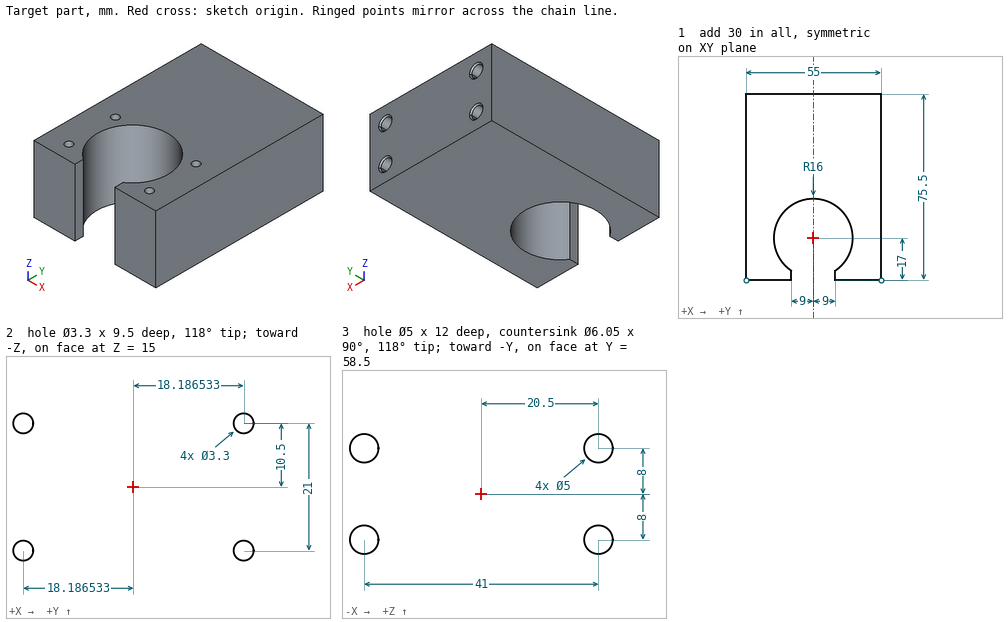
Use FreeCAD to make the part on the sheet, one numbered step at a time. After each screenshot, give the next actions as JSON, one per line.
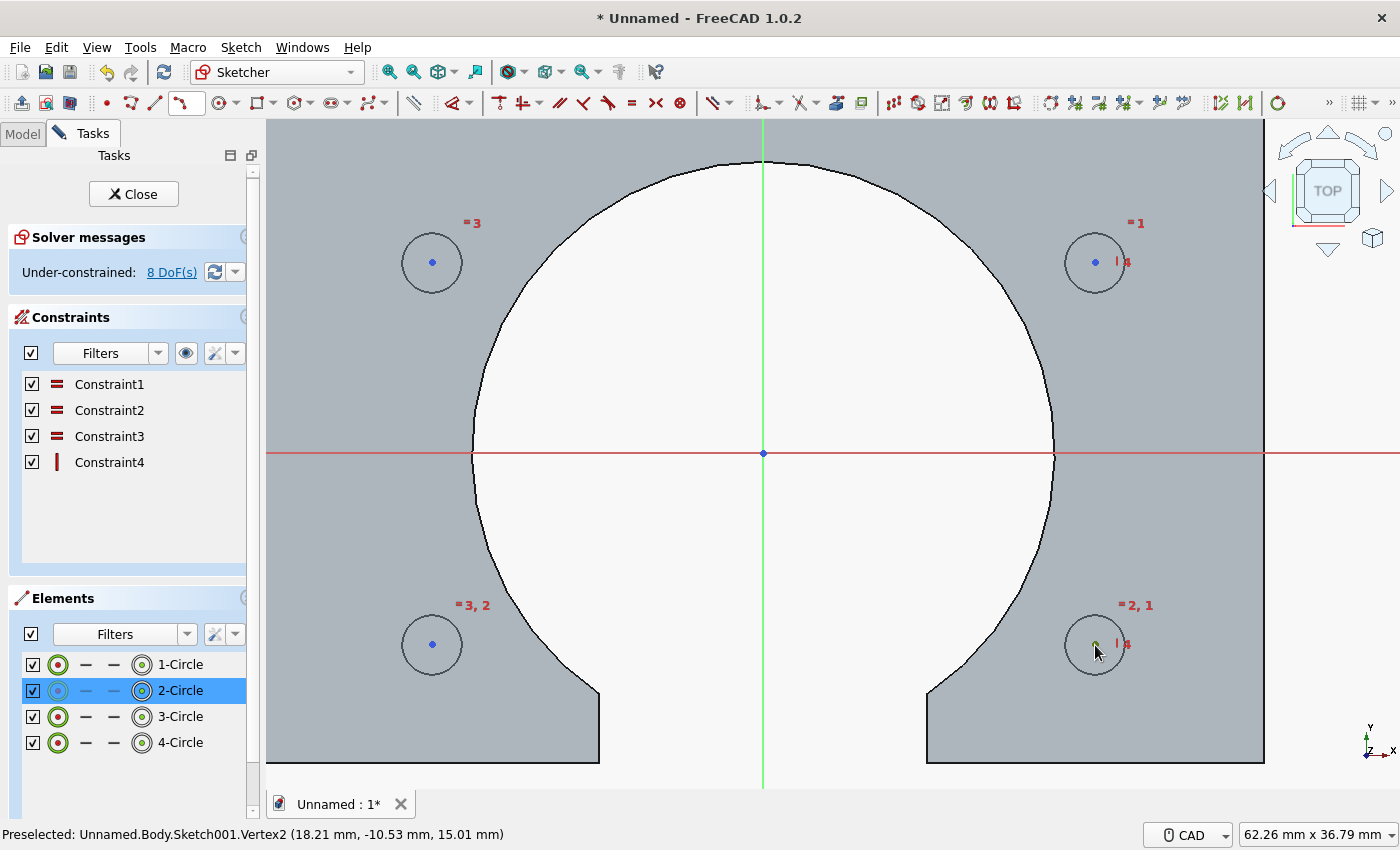
{"action": "left_click", "coordinate": [432, 645]}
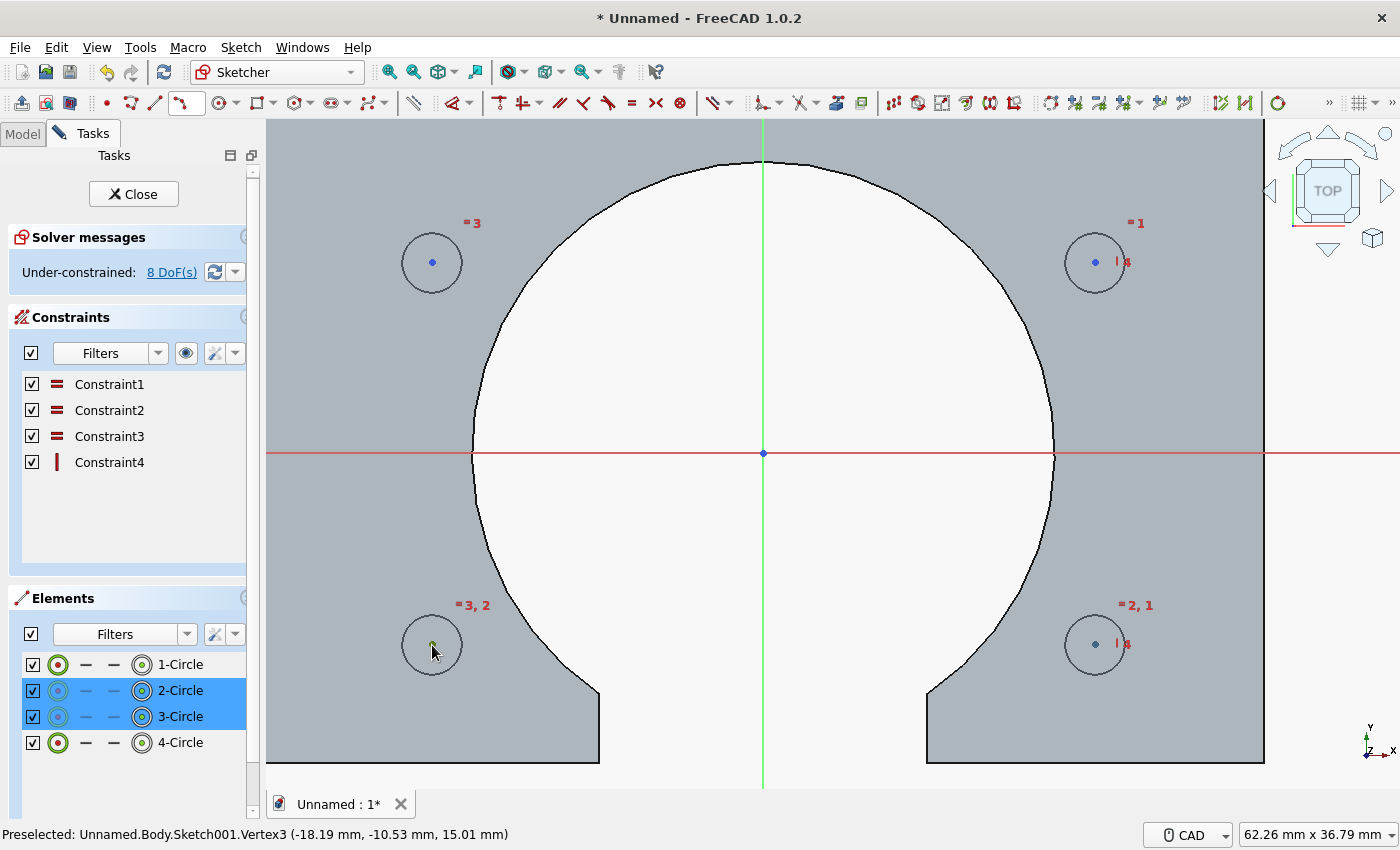
{"action": "left_click", "coordinate": [542, 104]}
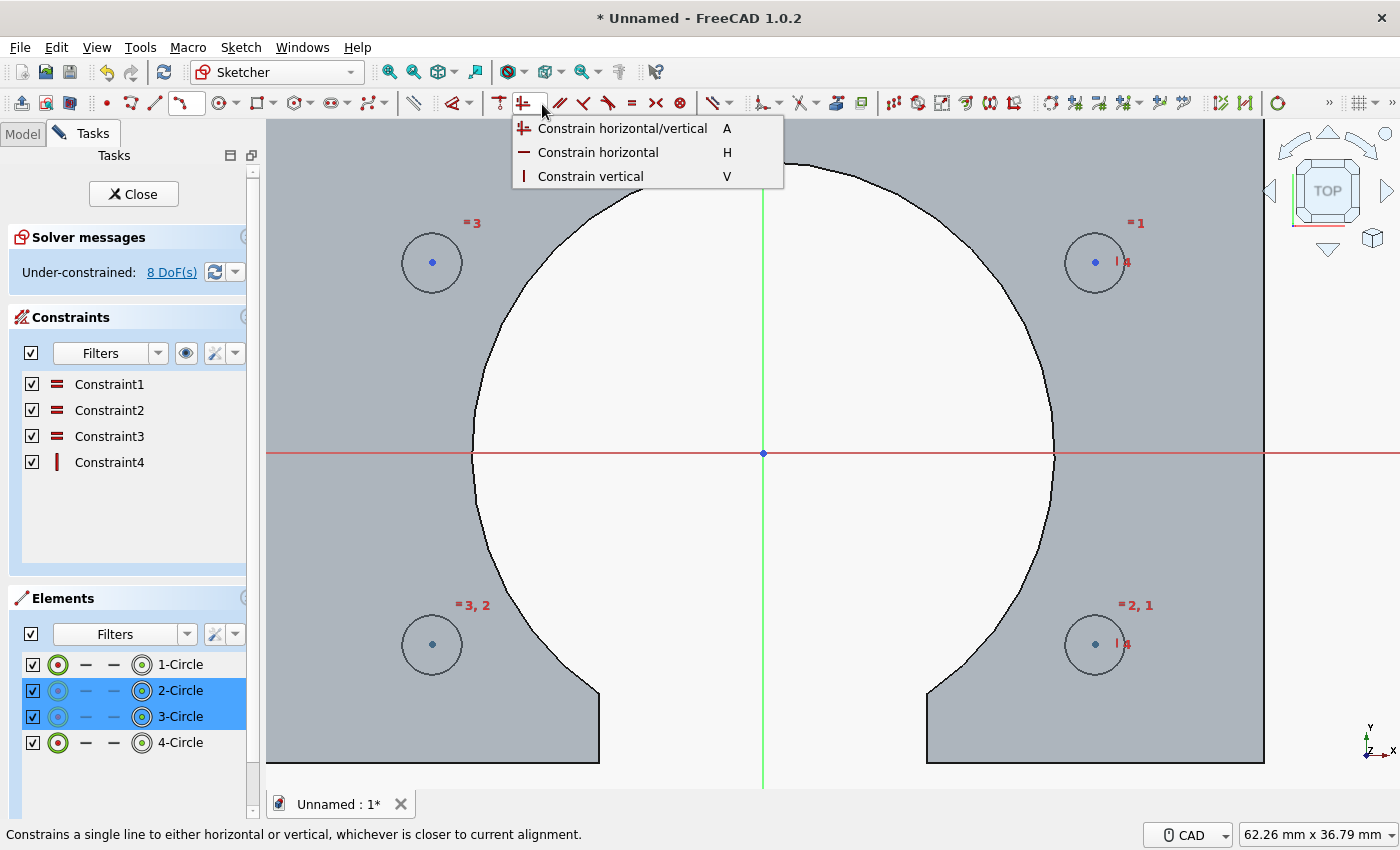
{"action": "left_click", "coordinate": [648, 152]}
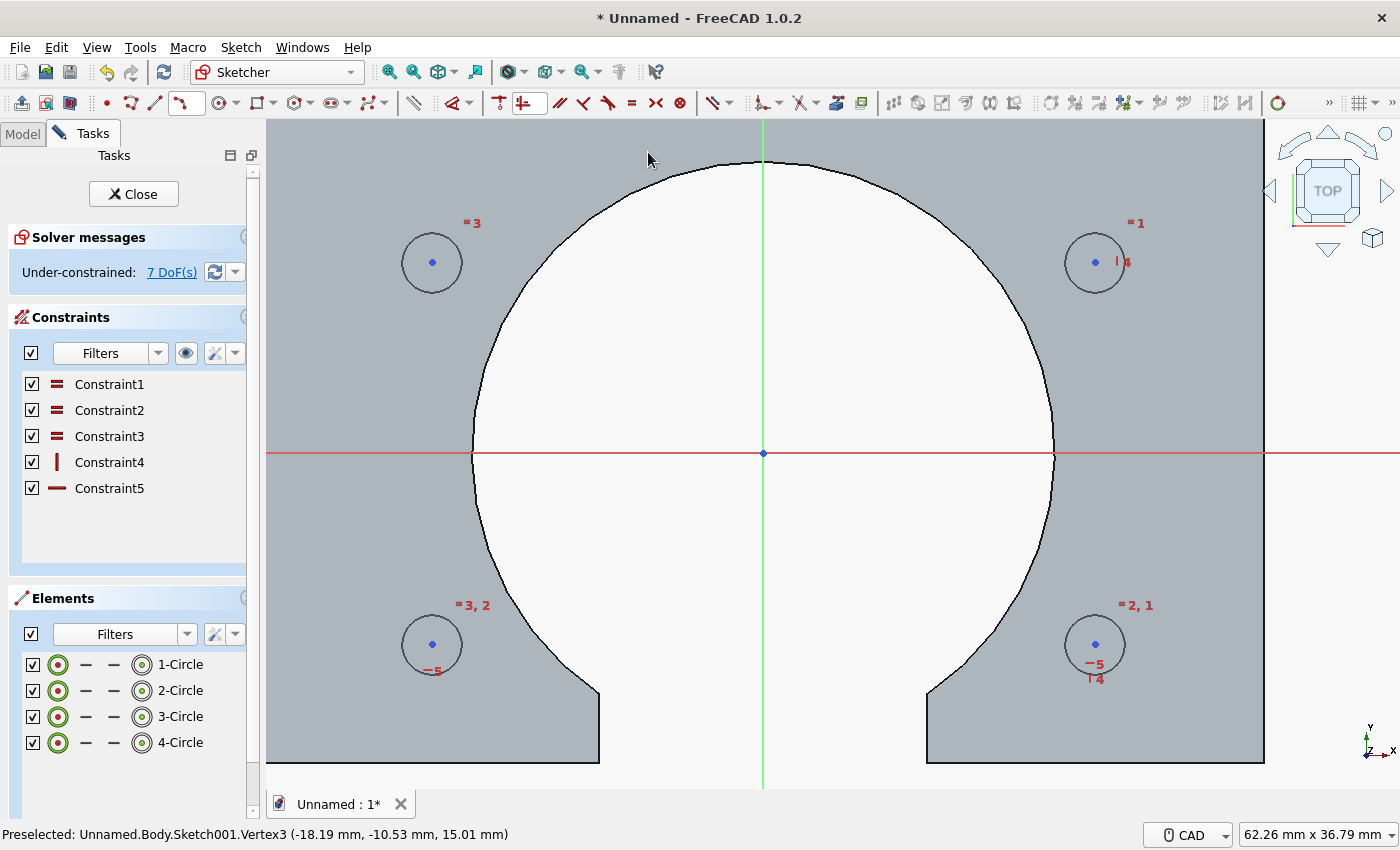
{"action": "left_click", "coordinate": [432, 645]}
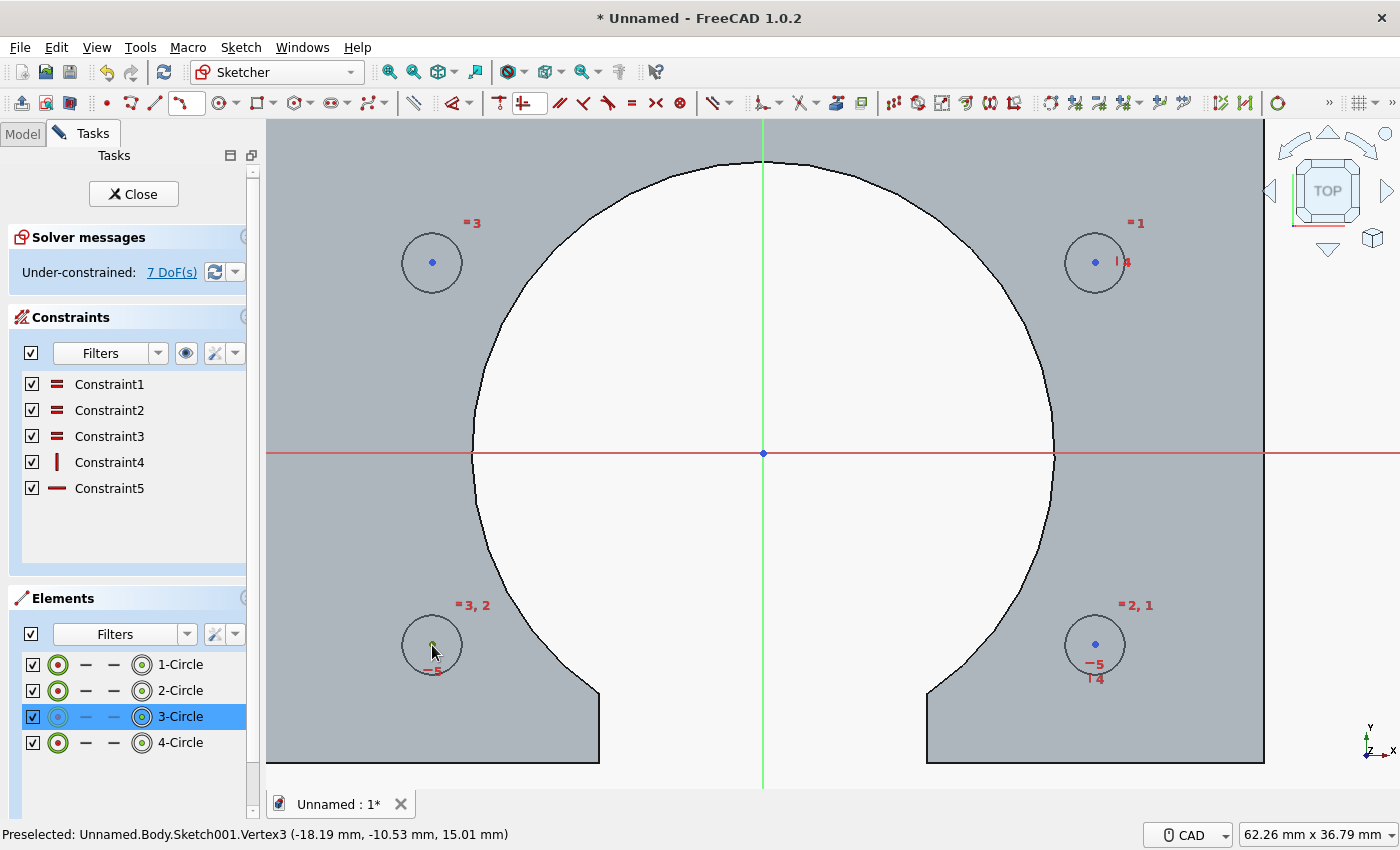
{"action": "left_click", "coordinate": [432, 263]}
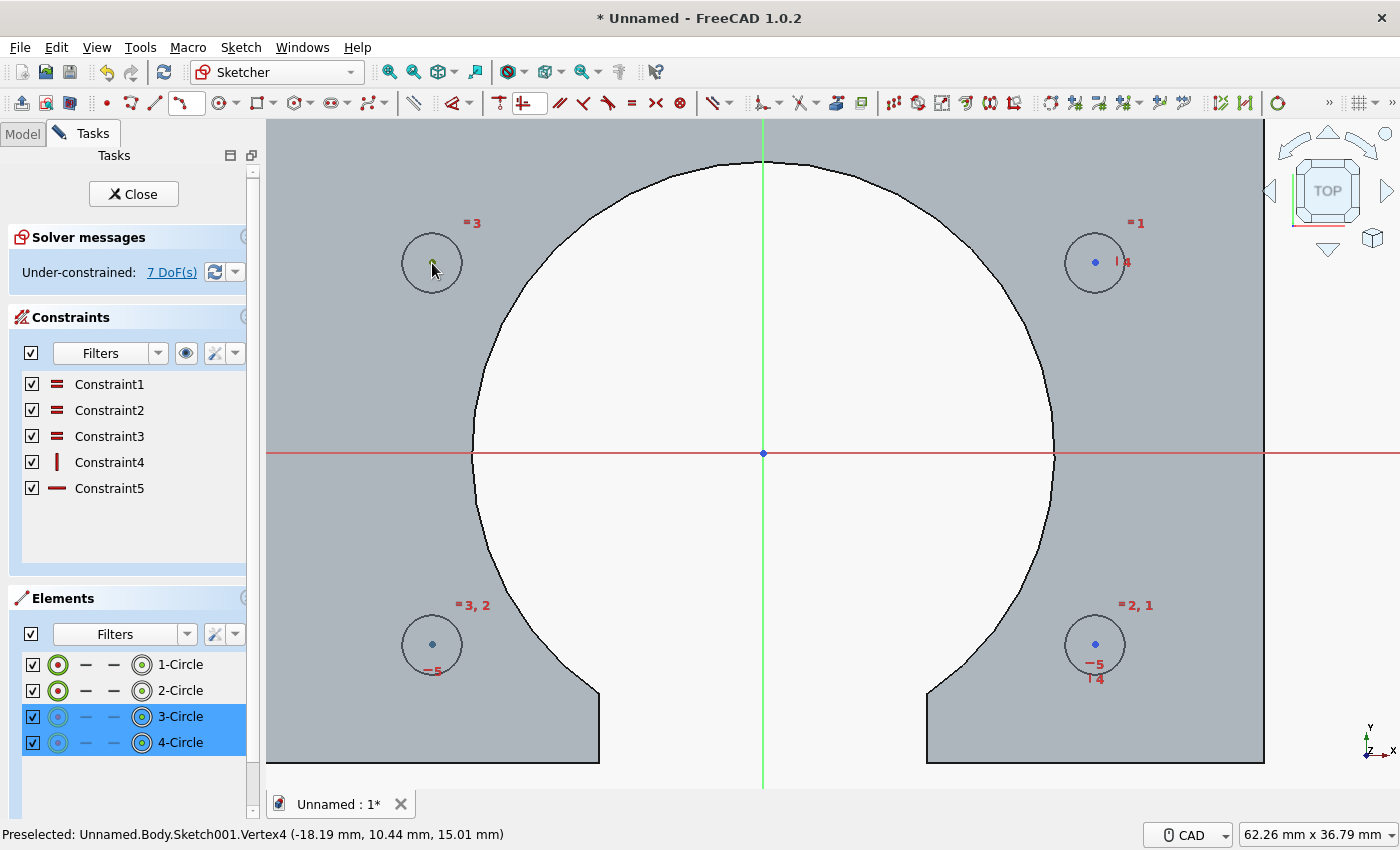
{"action": "left_click", "coordinate": [542, 104]}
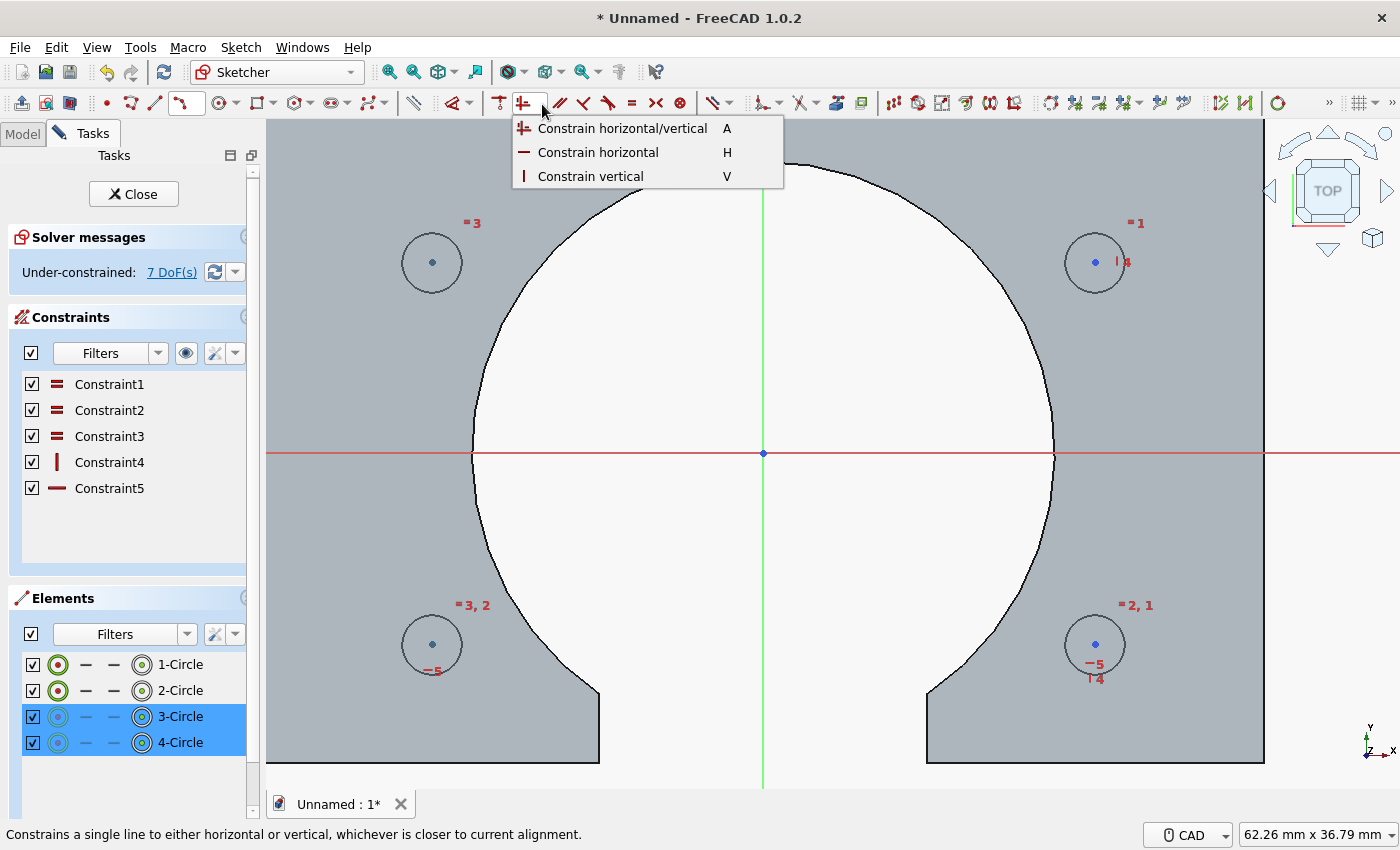
{"action": "left_click", "coordinate": [648, 176]}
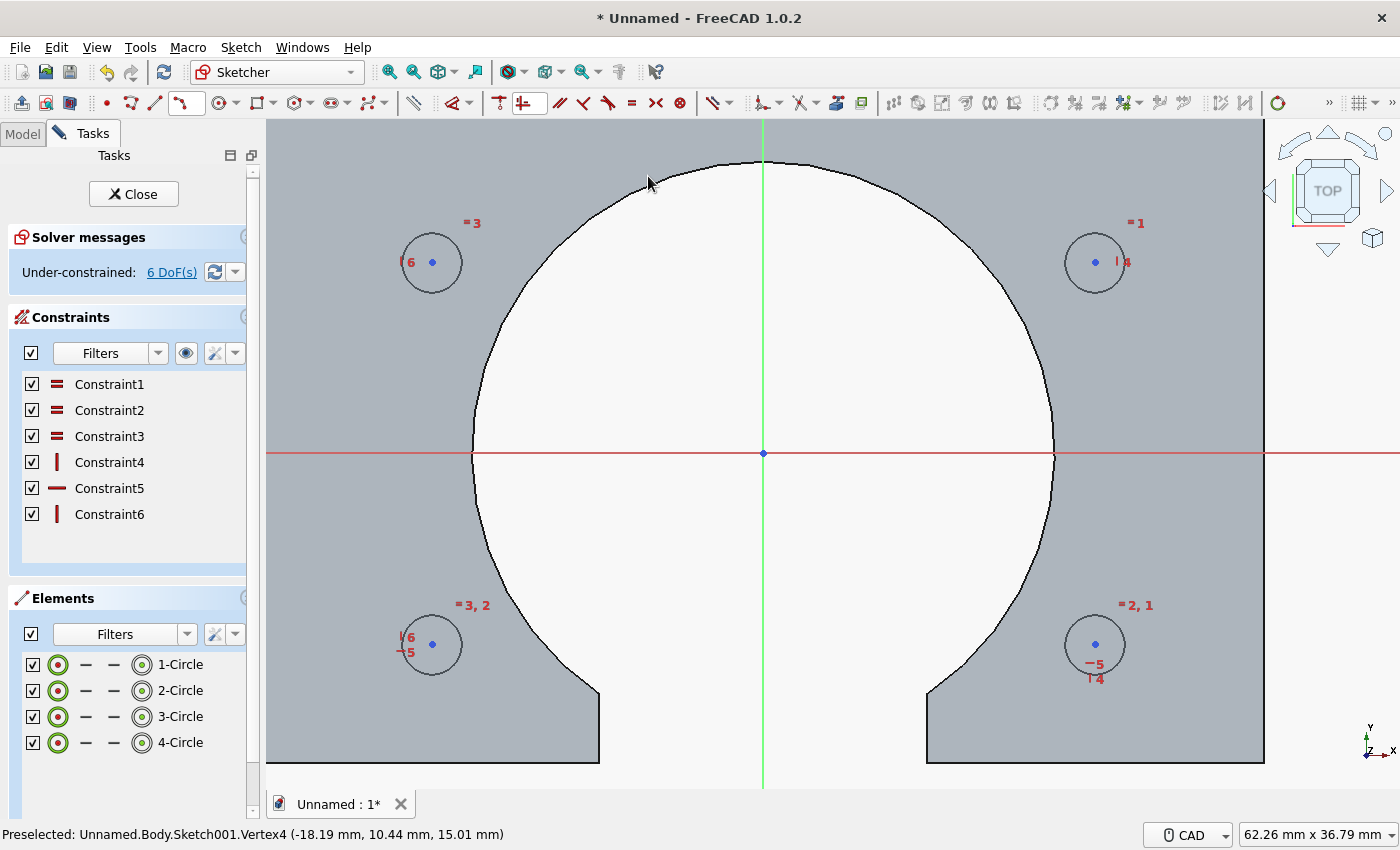
{"action": "left_click", "coordinate": [1095, 263]}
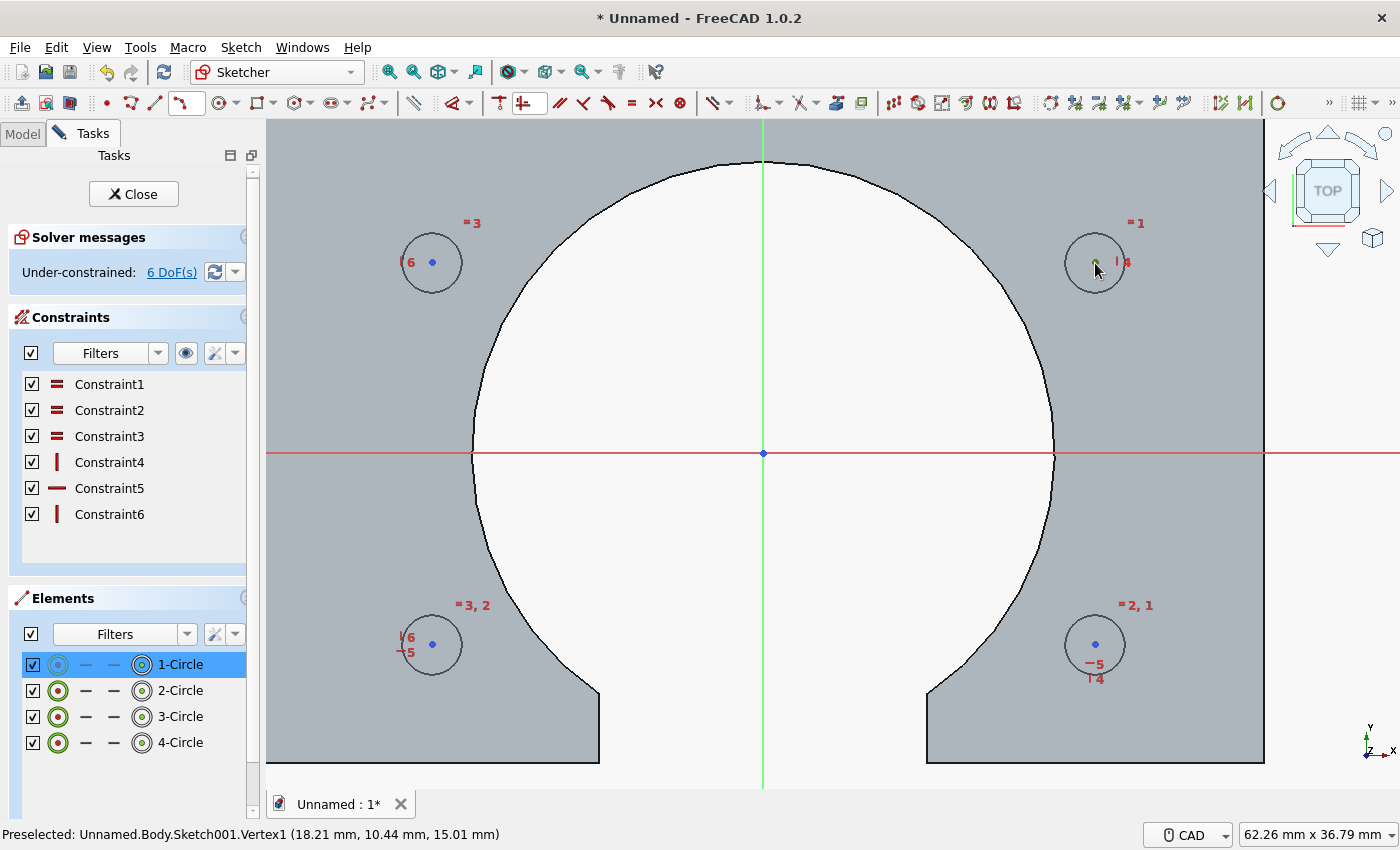
{"action": "left_click", "coordinate": [432, 263]}